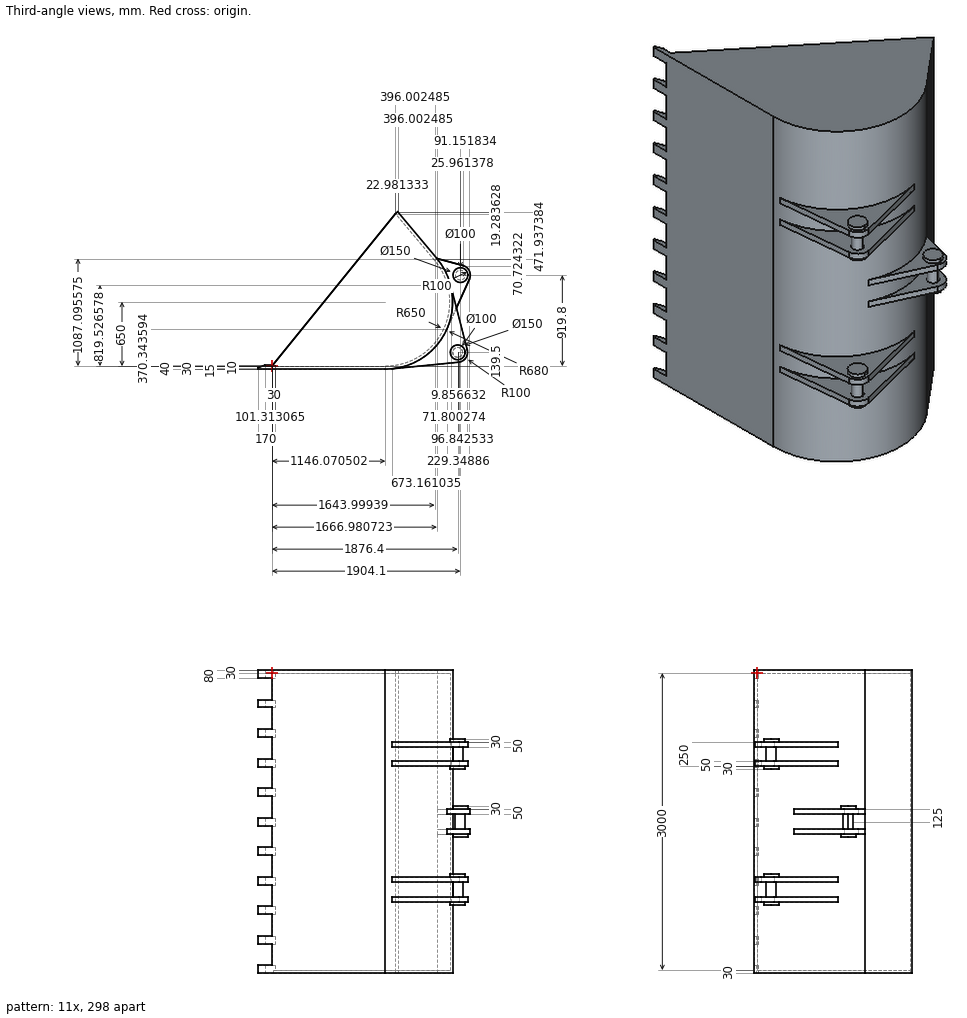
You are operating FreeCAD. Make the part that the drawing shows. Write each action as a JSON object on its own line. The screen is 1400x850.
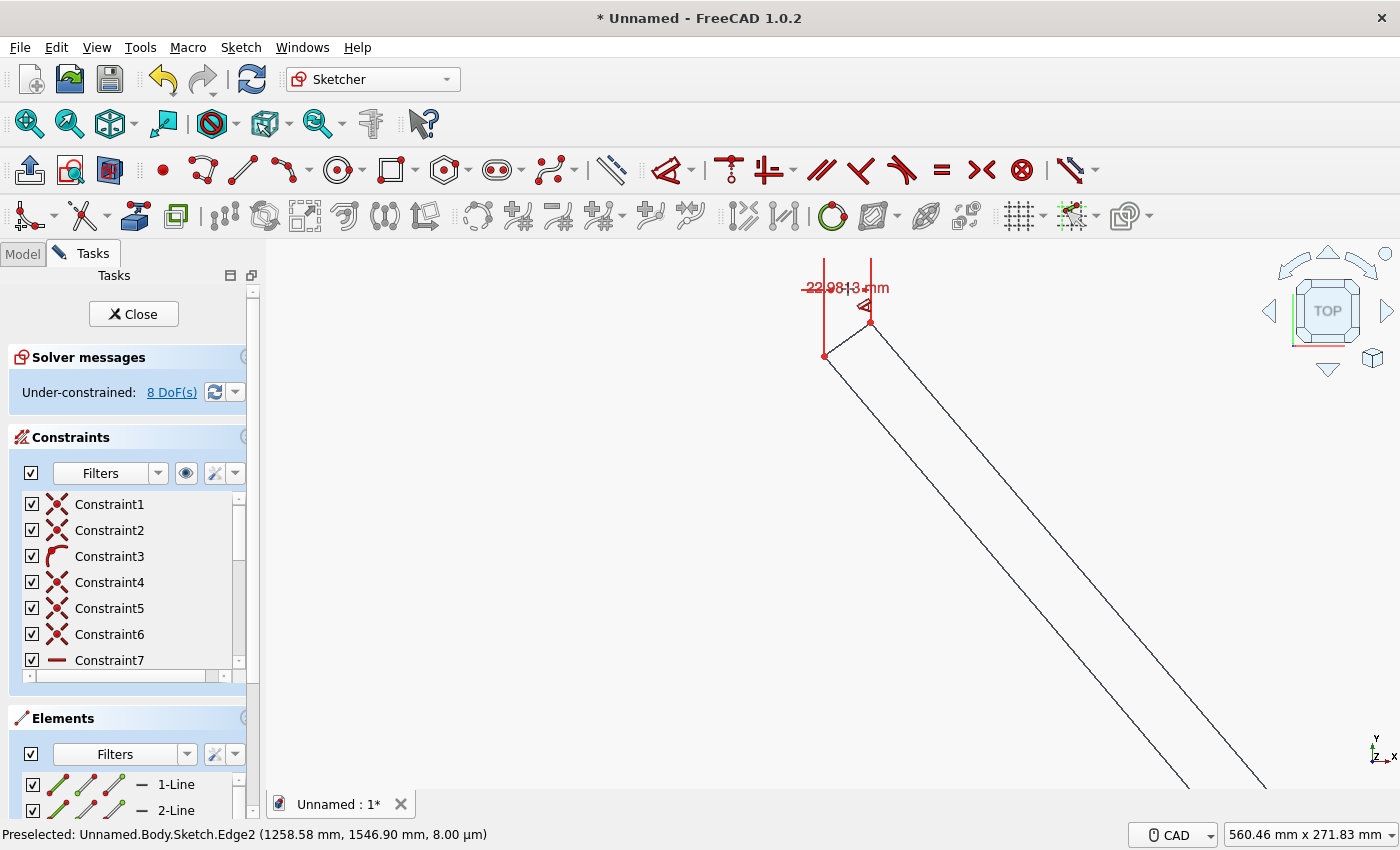
{"action": "left_click", "coordinate": [857, 333]}
{"action": "left_click", "coordinate": [905, 340]}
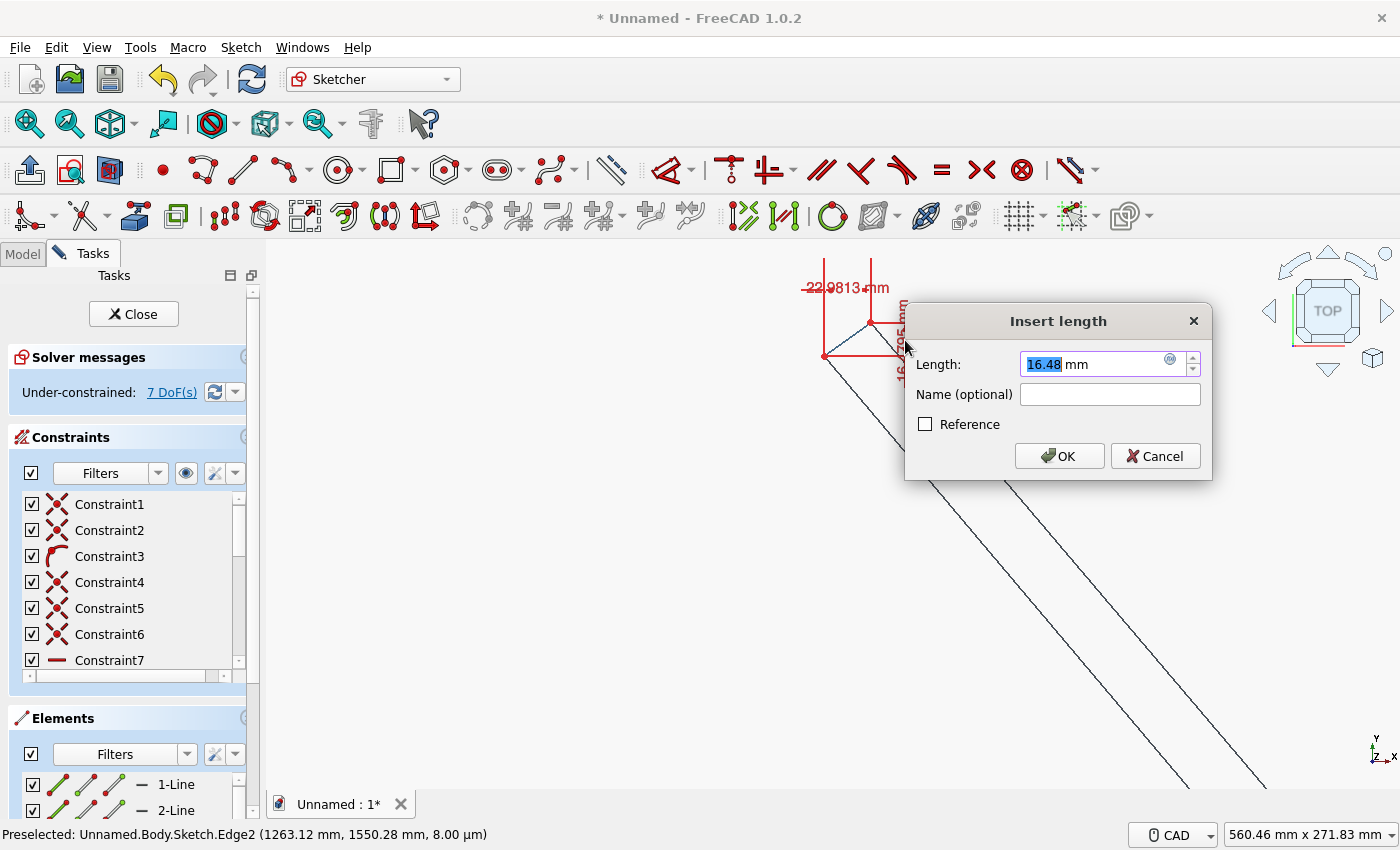
{"action": "type", "text": "19.283628"}
{"action": "key", "text": "Return"}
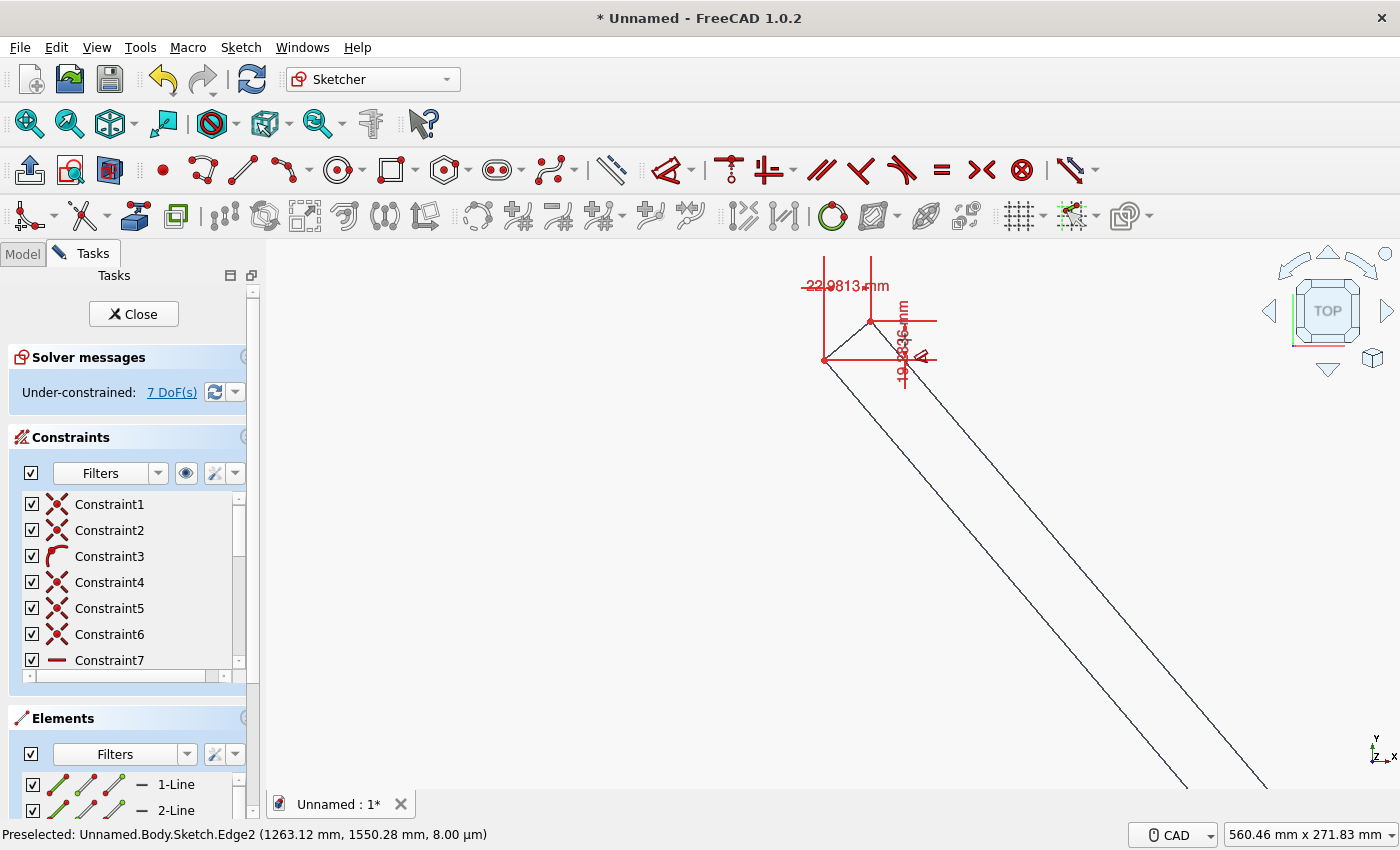
{"action": "scroll", "coordinate": [849, 338], "scroll_direction": "down", "scroll_amount": 11}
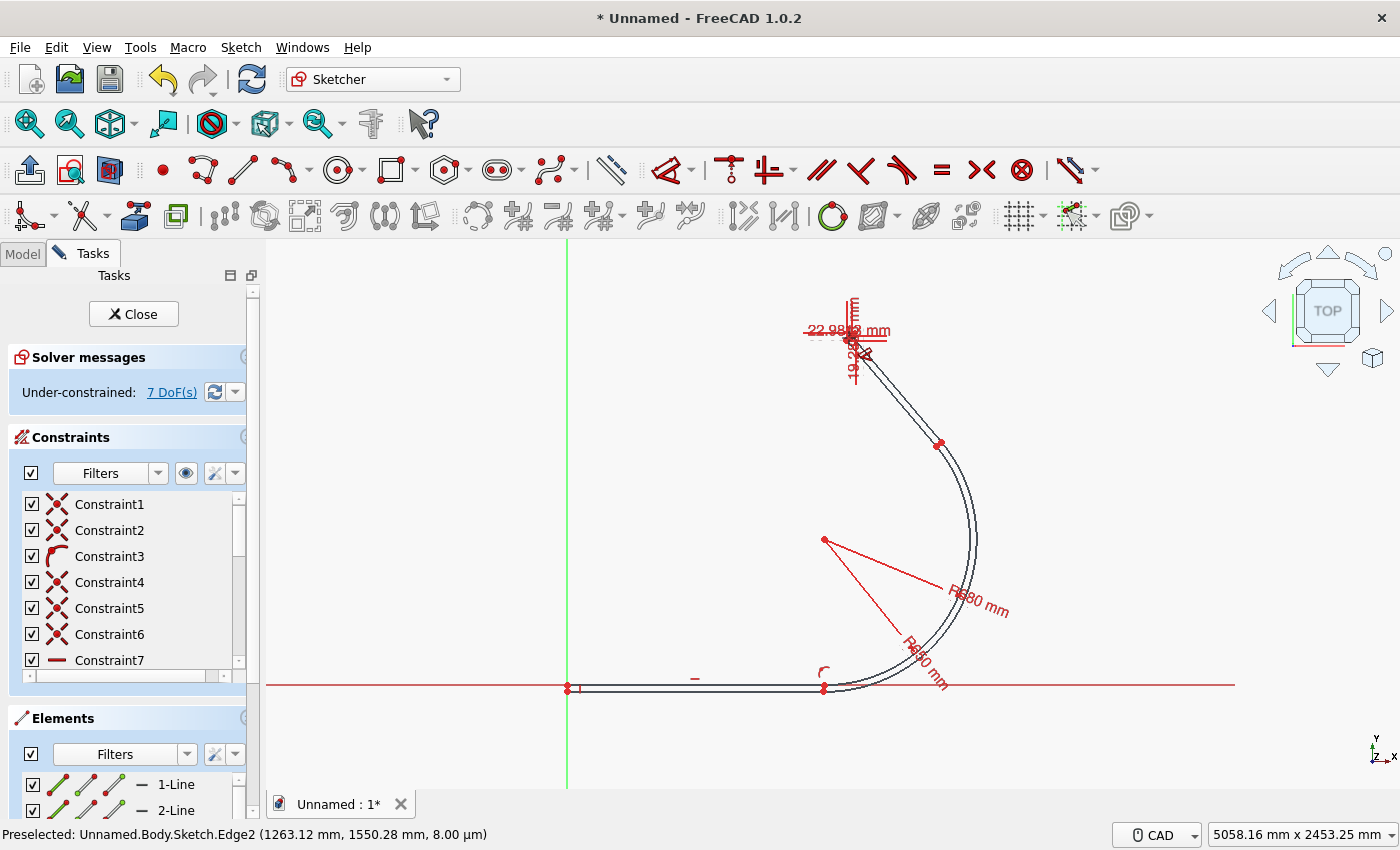
{"action": "scroll", "coordinate": [747, 685], "scroll_direction": "up", "scroll_amount": 4}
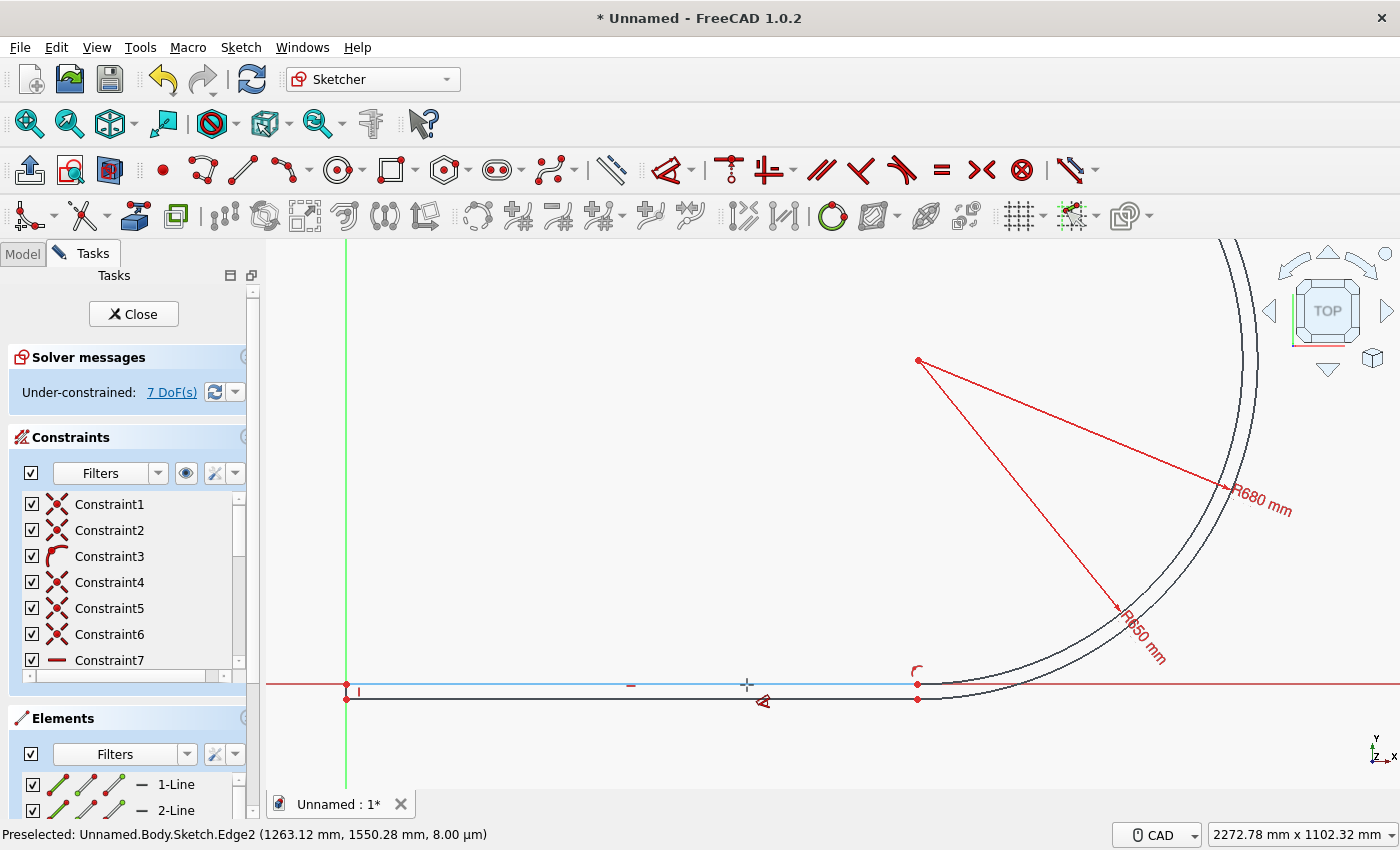
{"action": "left_click", "coordinate": [746, 684]}
{"action": "left_click", "coordinate": [632, 718]}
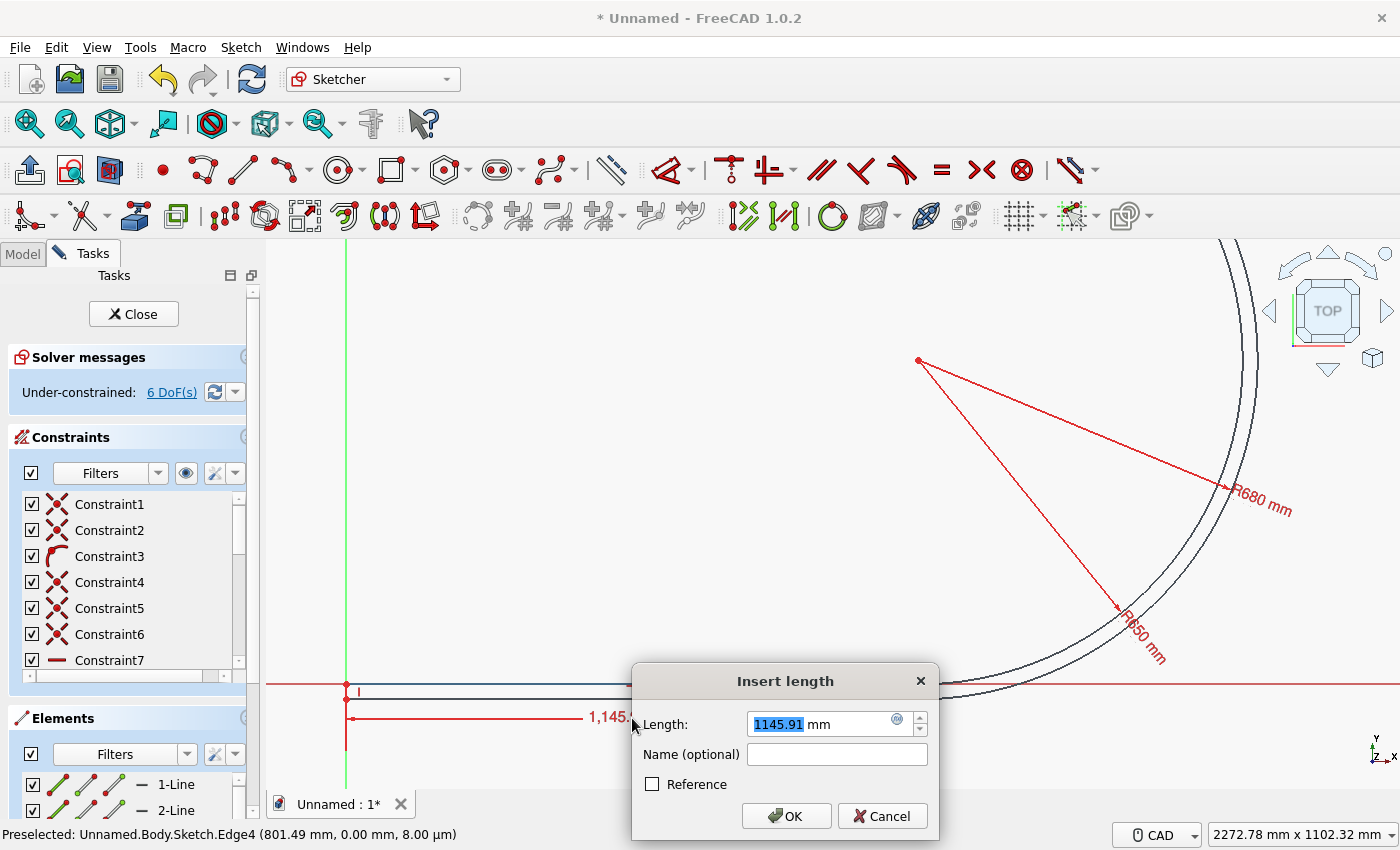
{"action": "type", "text": "1146.070502"}
{"action": "key", "text": "Return"}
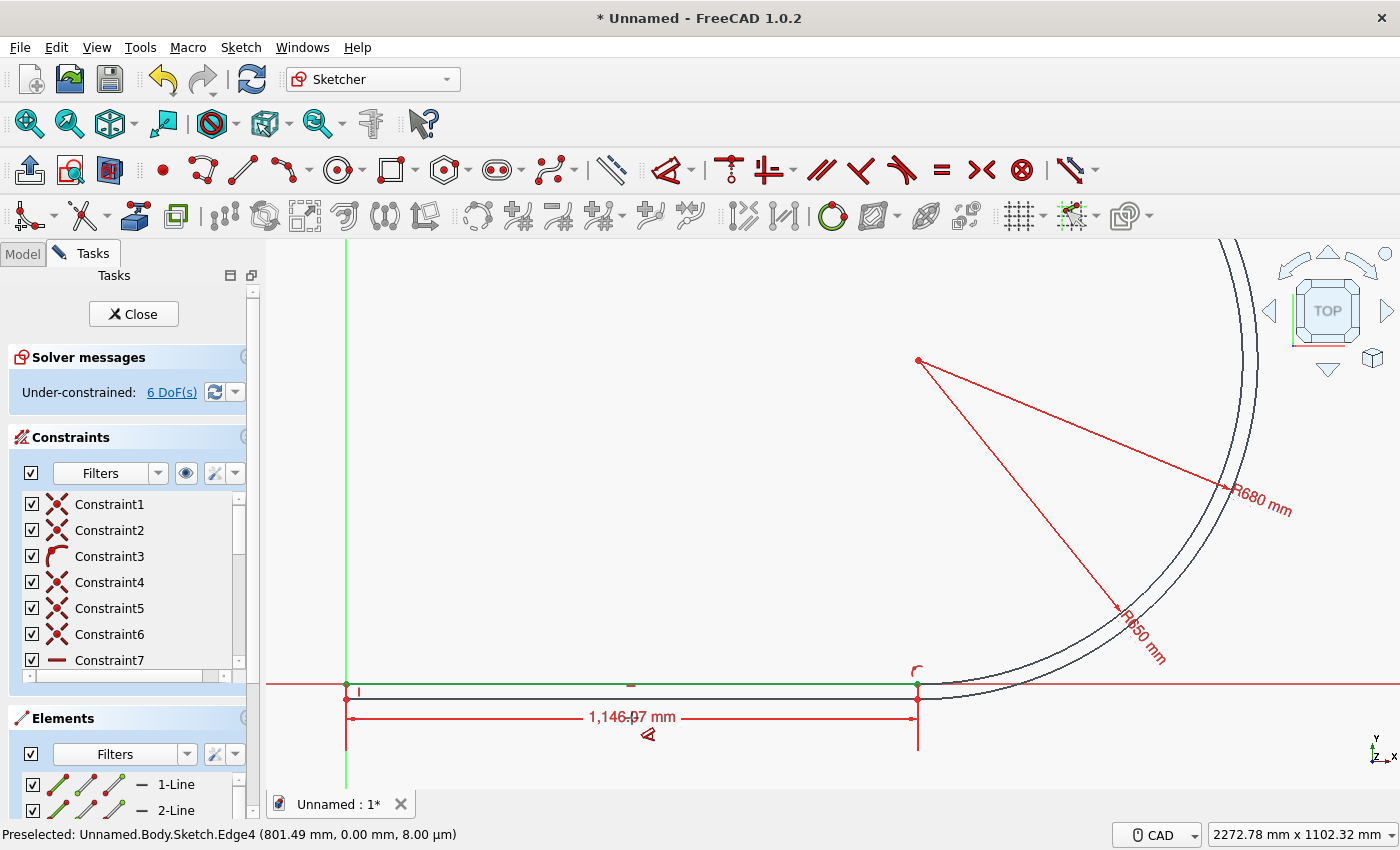
{"action": "left_click", "coordinate": [518, 699]}
{"action": "left_click", "coordinate": [500, 733]}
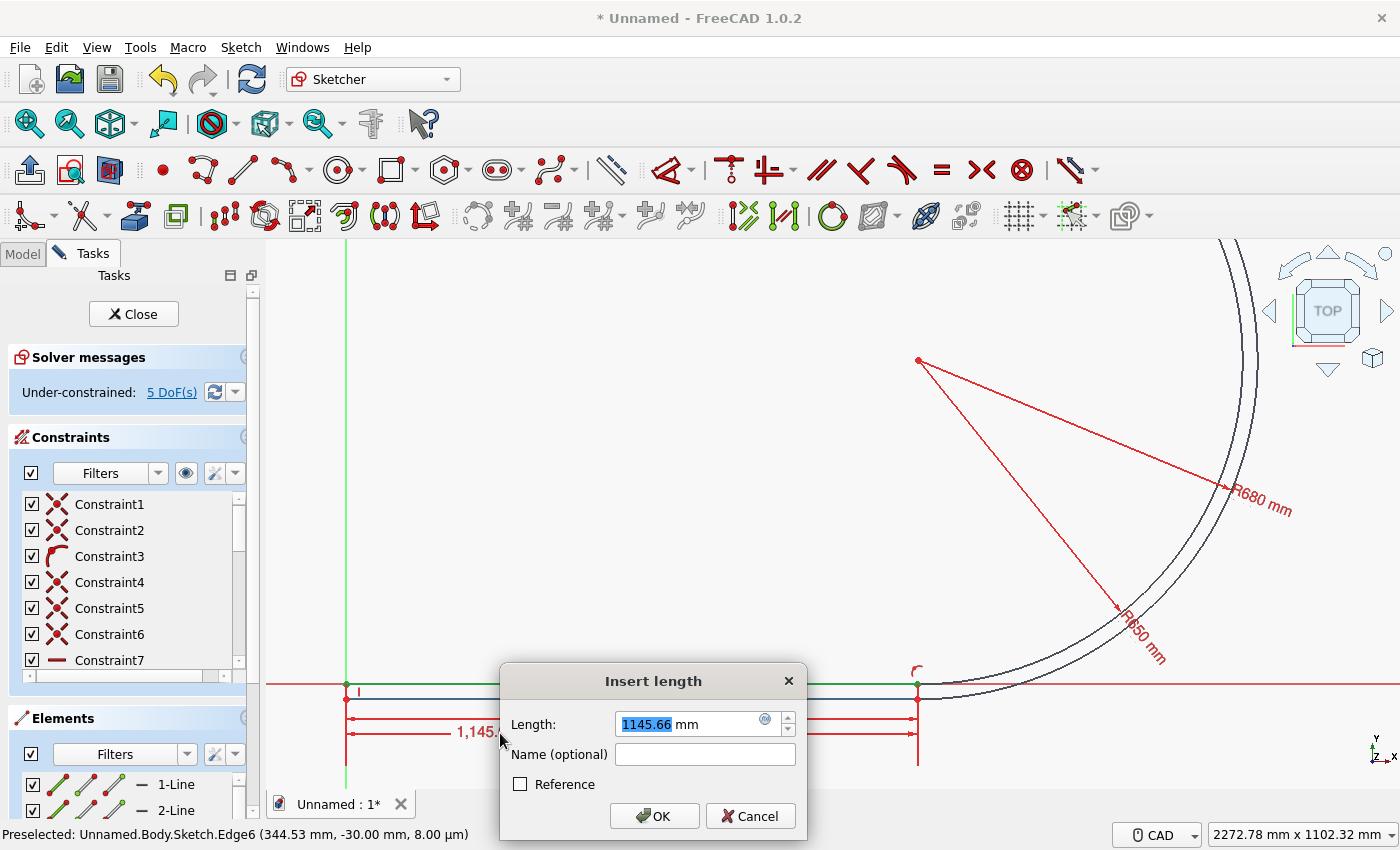
{"action": "type", "text": "1146.070502"}
{"action": "key", "text": "Return"}